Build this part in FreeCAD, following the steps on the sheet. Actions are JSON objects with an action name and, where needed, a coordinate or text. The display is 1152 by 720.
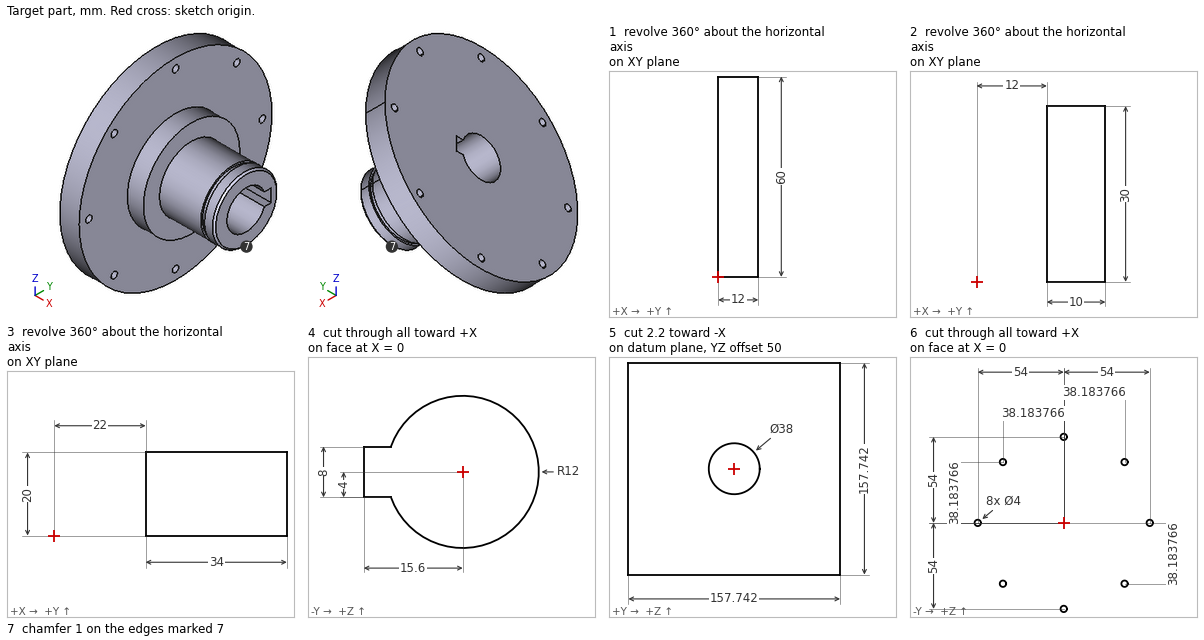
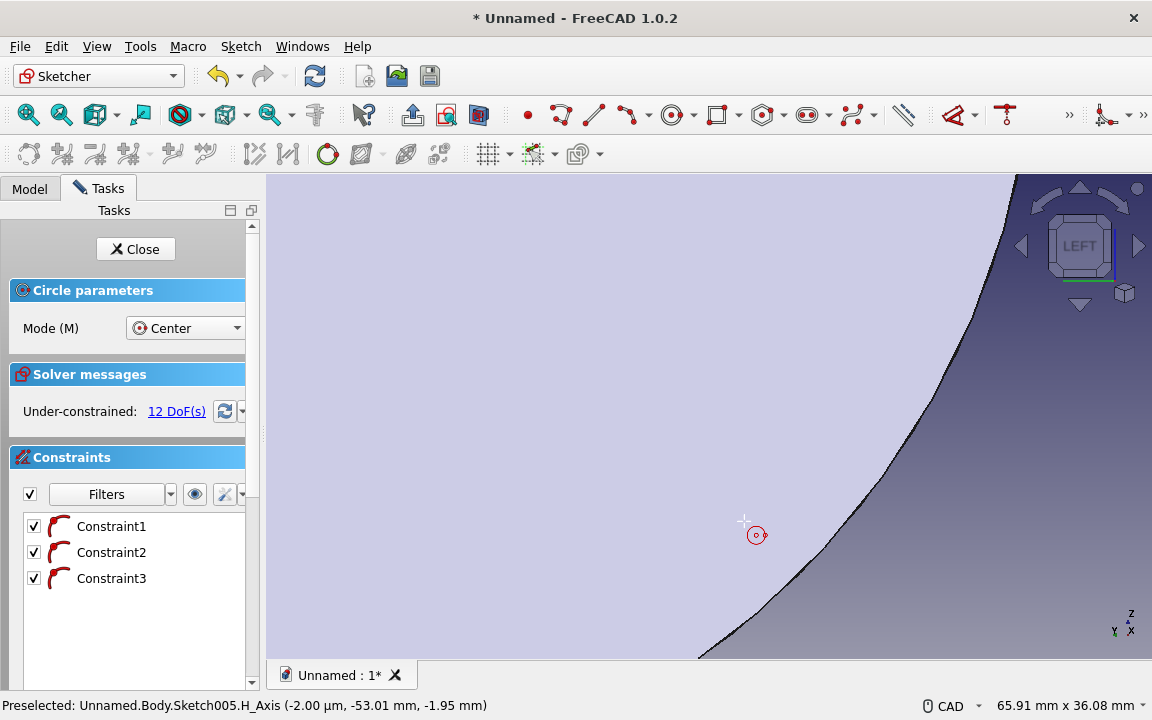
{"action": "scroll", "coordinate": [744, 521], "scroll_direction": "down", "scroll_amount": 8}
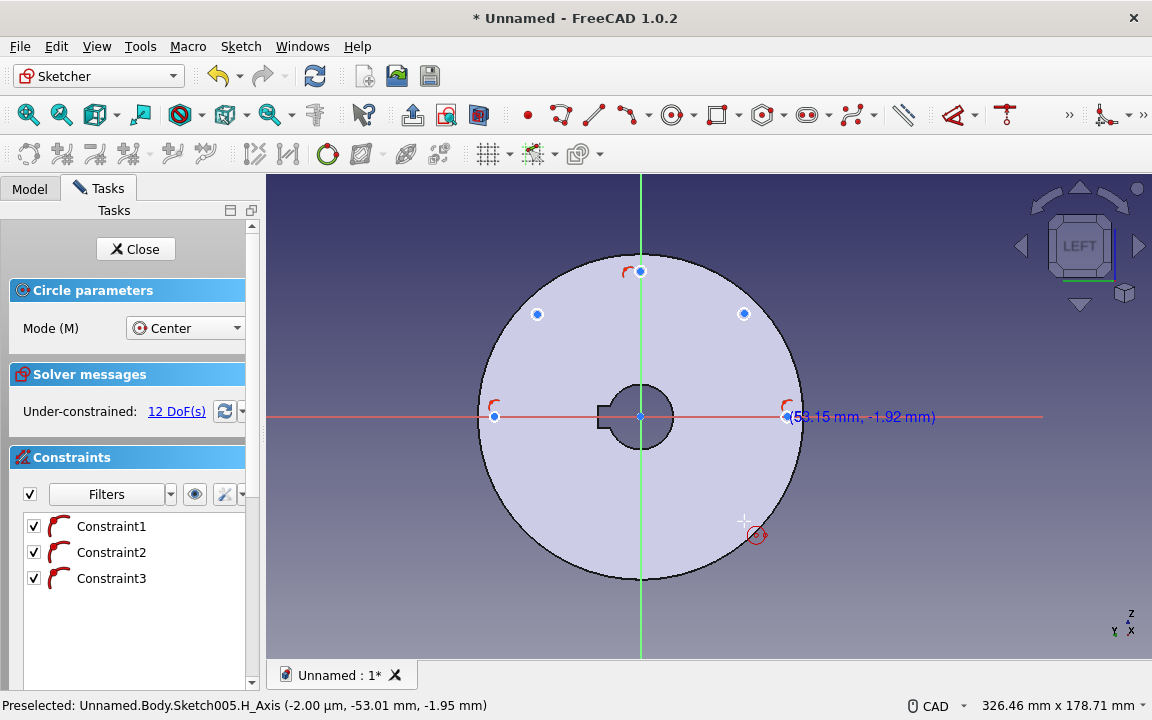
{"action": "left_click", "coordinate": [744, 521]}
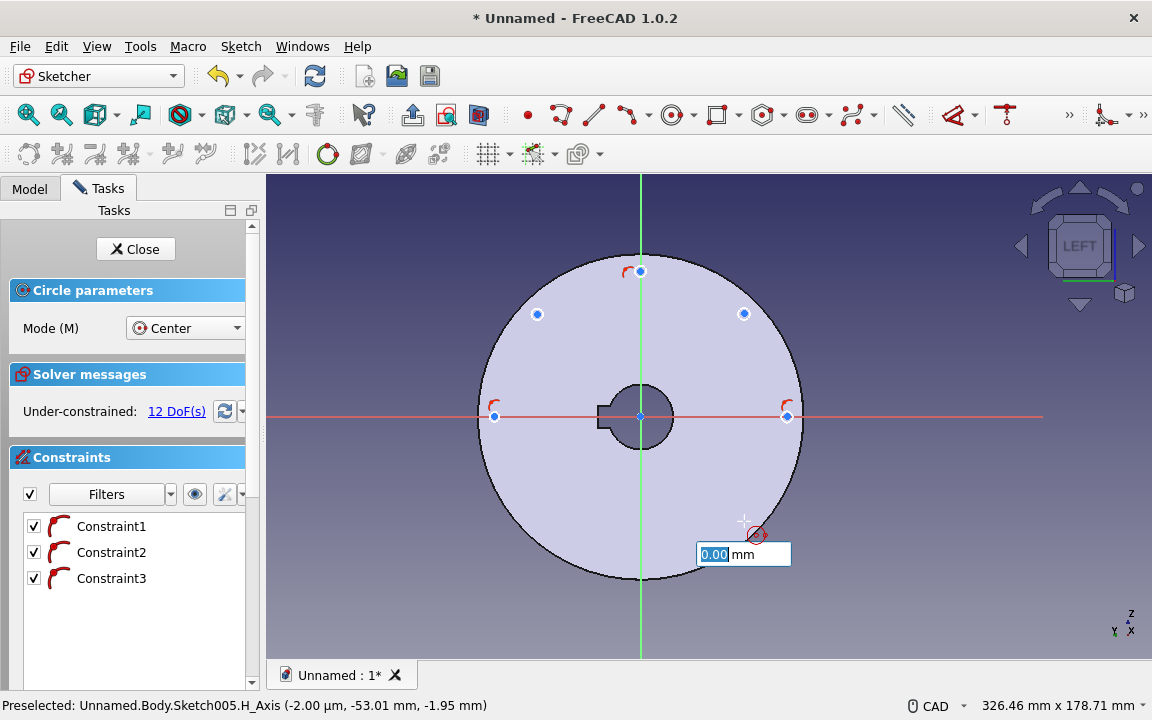
{"action": "scroll", "coordinate": [748, 517], "scroll_direction": "up", "scroll_amount": 6}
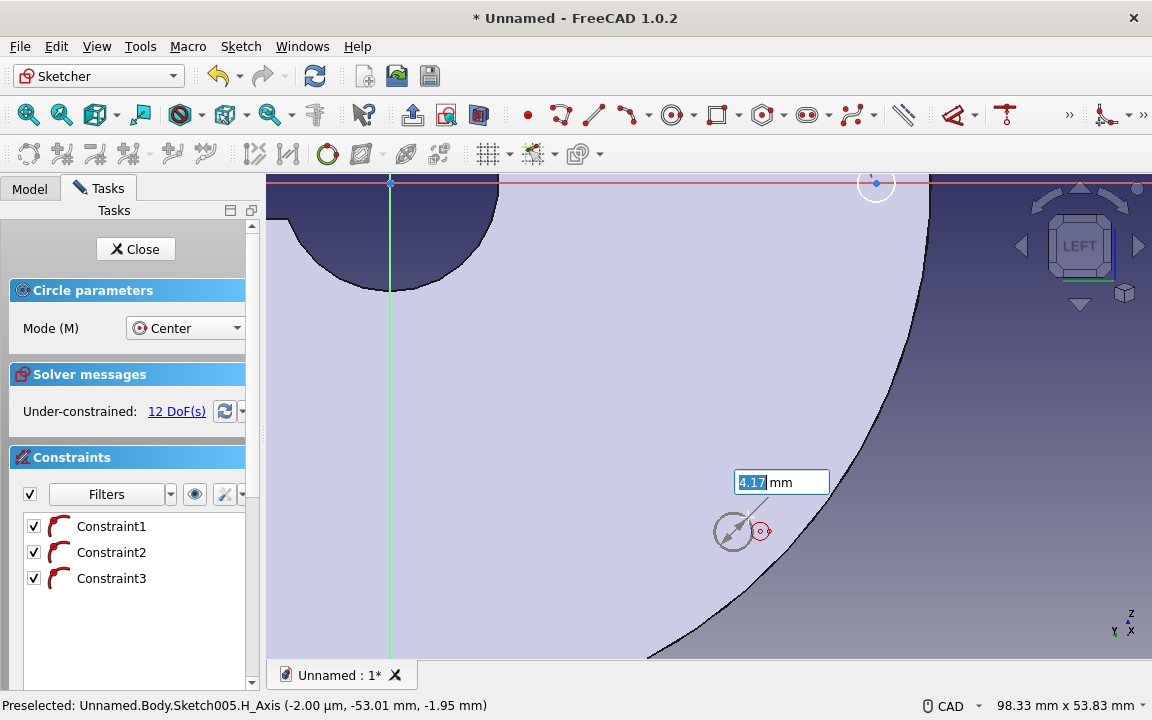
{"action": "left_click", "coordinate": [747, 515]}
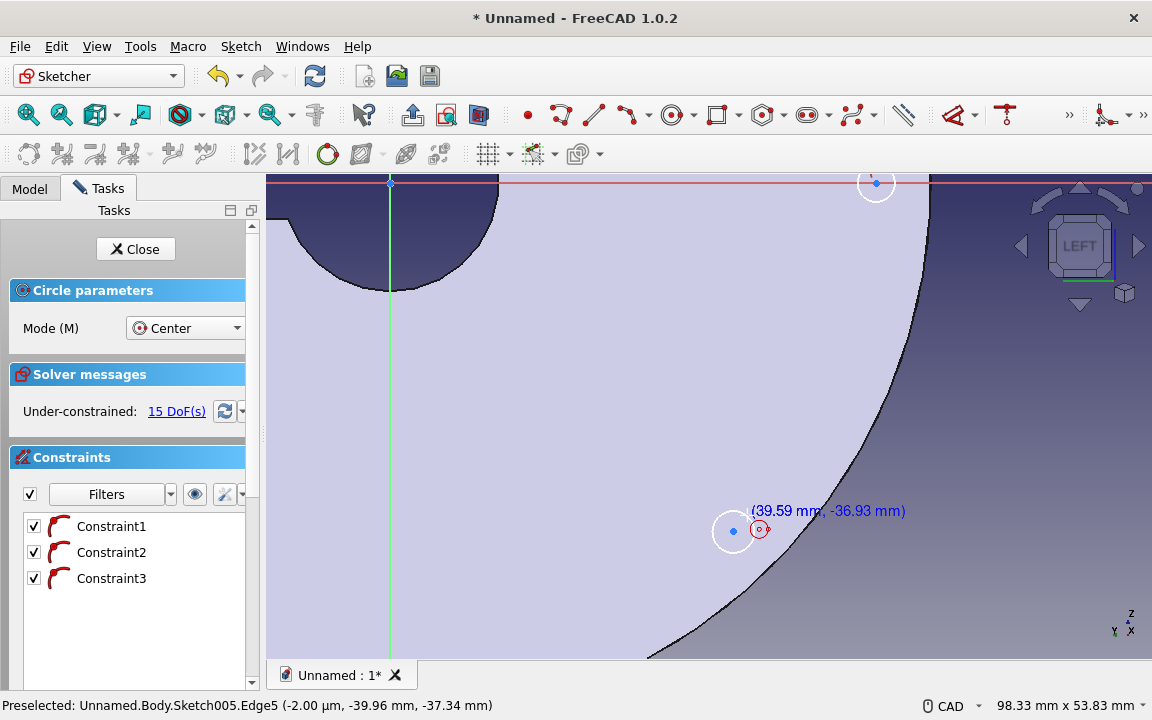
{"action": "scroll", "coordinate": [748, 517], "scroll_direction": "down", "scroll_amount": 6}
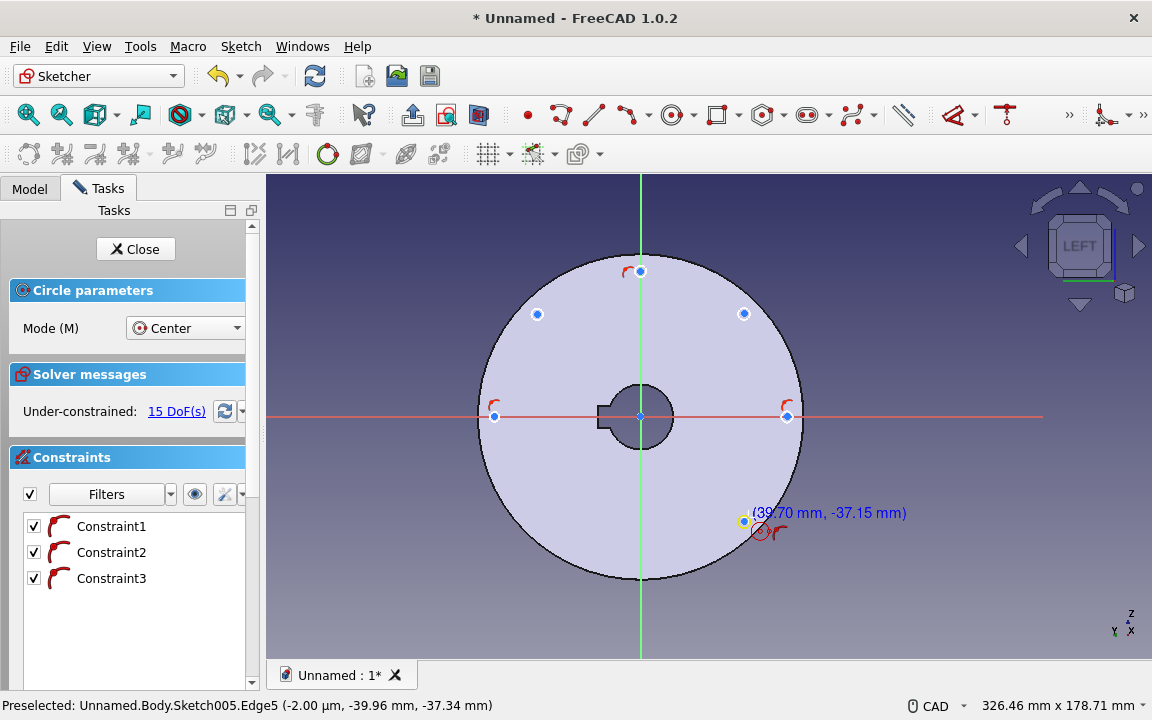
{"action": "scroll", "coordinate": [641, 564], "scroll_direction": "up", "scroll_amount": 8}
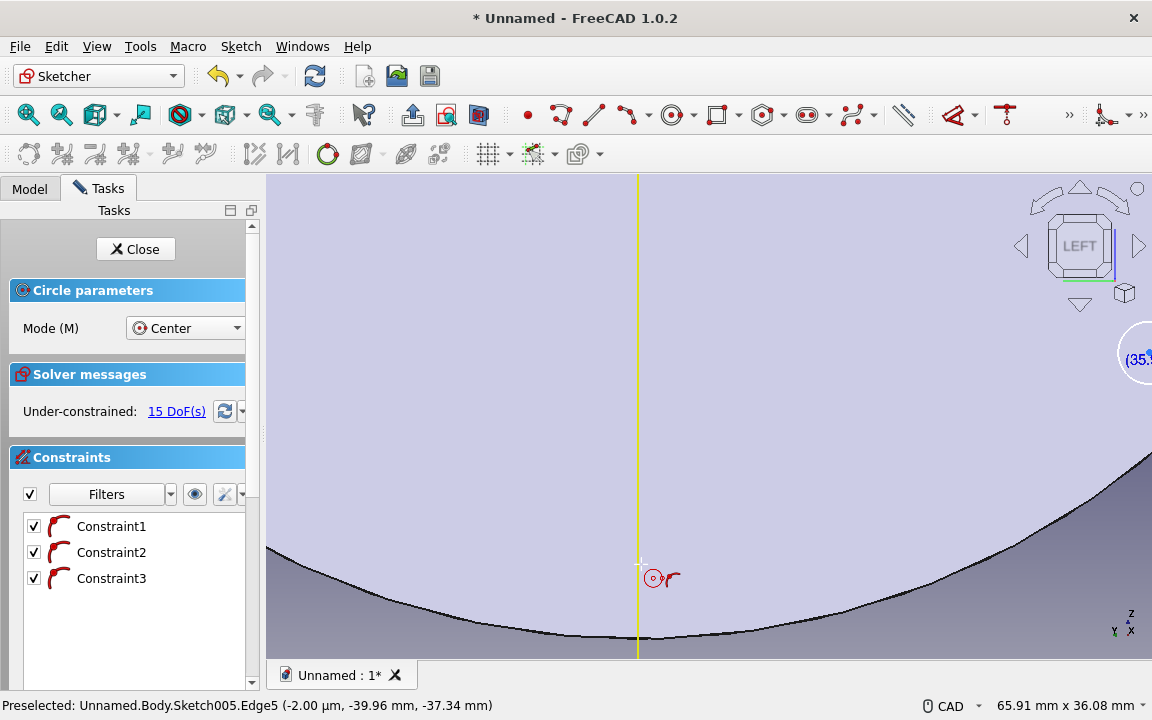
{"action": "scroll", "coordinate": [641, 564], "scroll_direction": "down", "scroll_amount": 8}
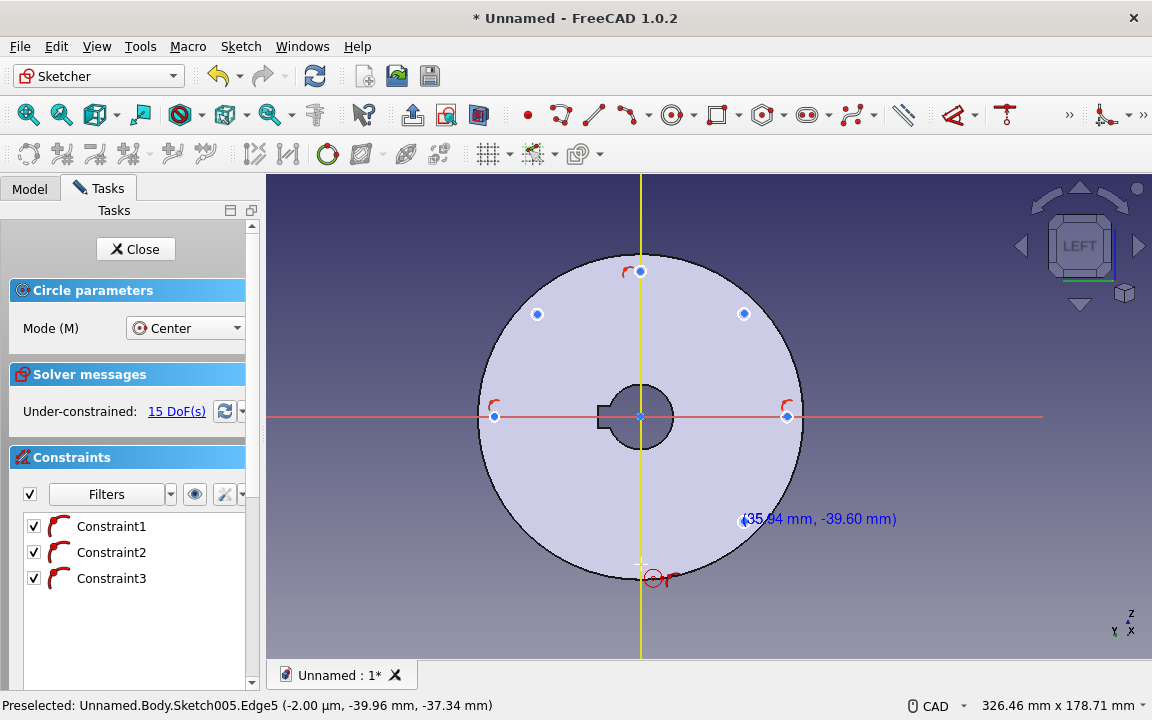
{"action": "left_click", "coordinate": [641, 564]}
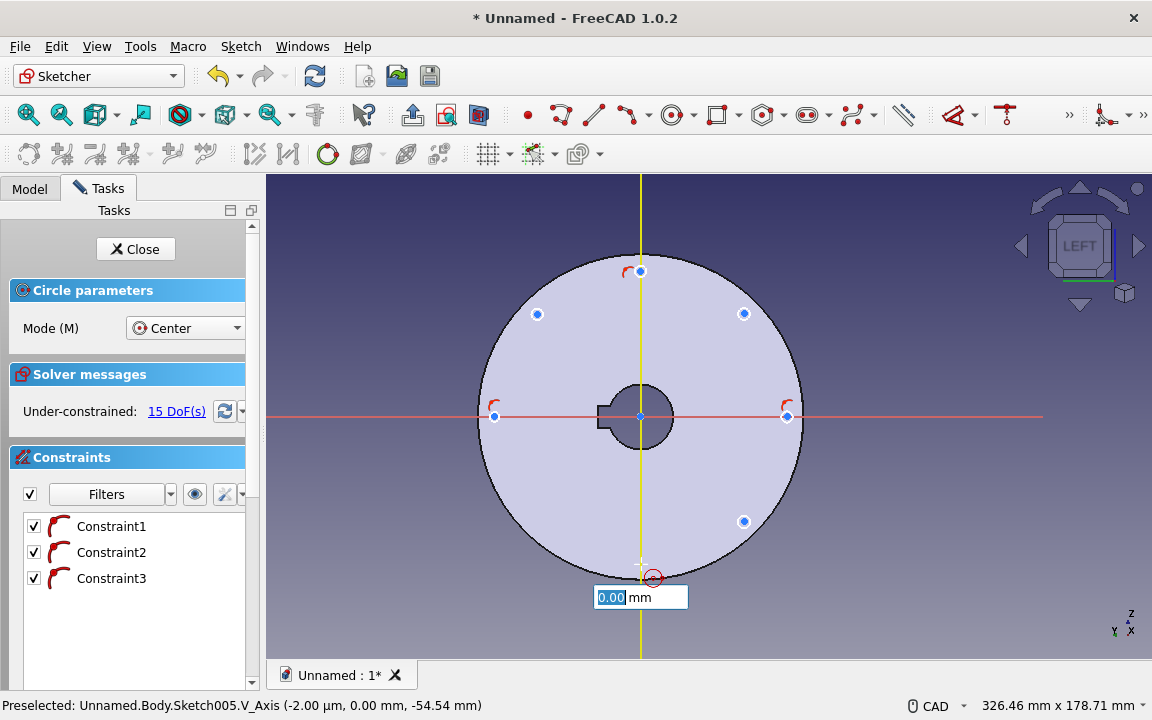
{"action": "scroll", "coordinate": [646, 562], "scroll_direction": "up", "scroll_amount": 6}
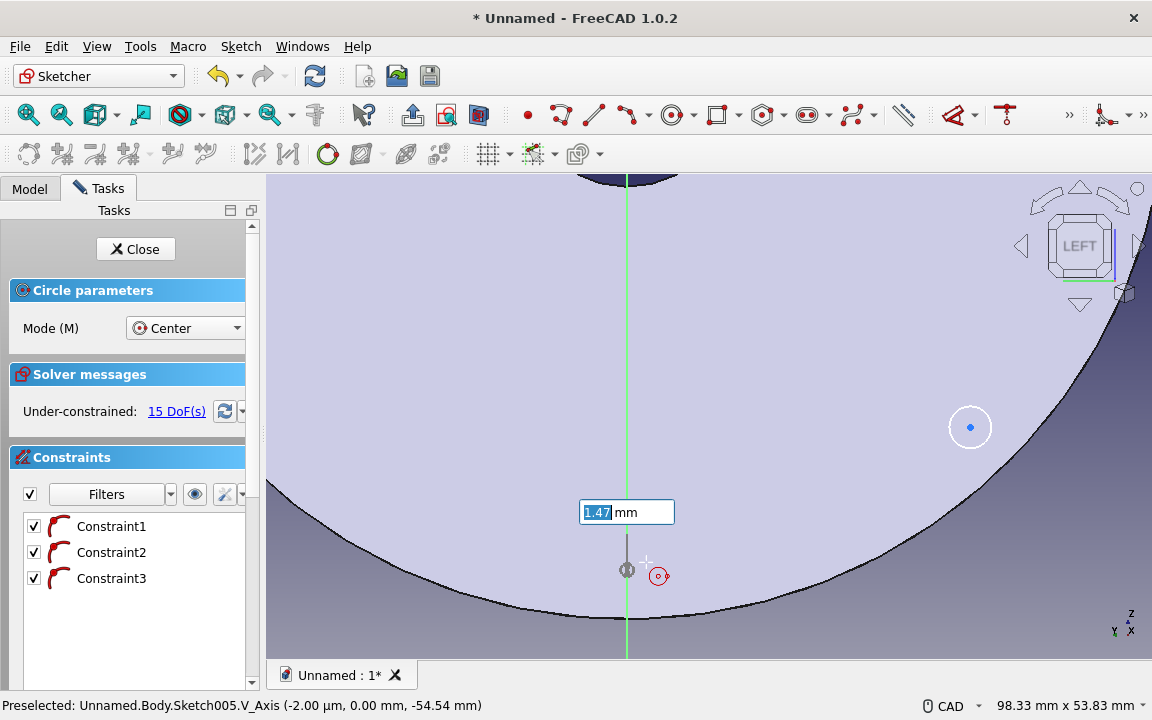
{"action": "left_click", "coordinate": [644, 559]}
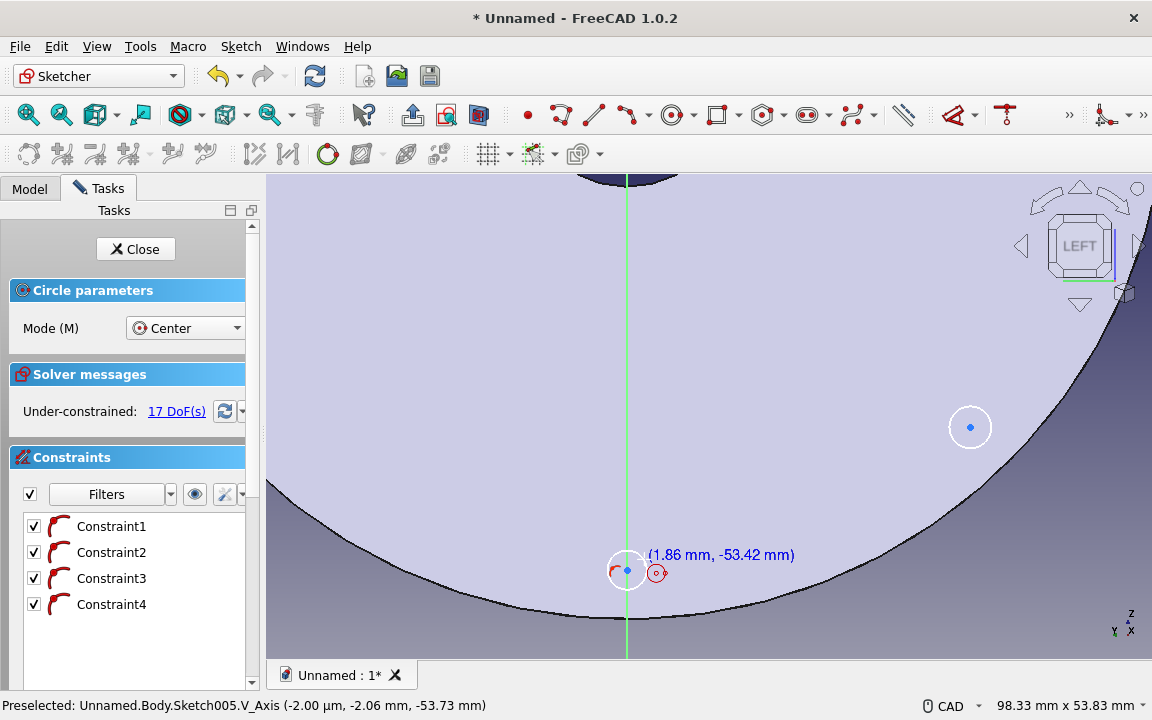
{"action": "scroll", "coordinate": [646, 562], "scroll_direction": "down", "scroll_amount": 6}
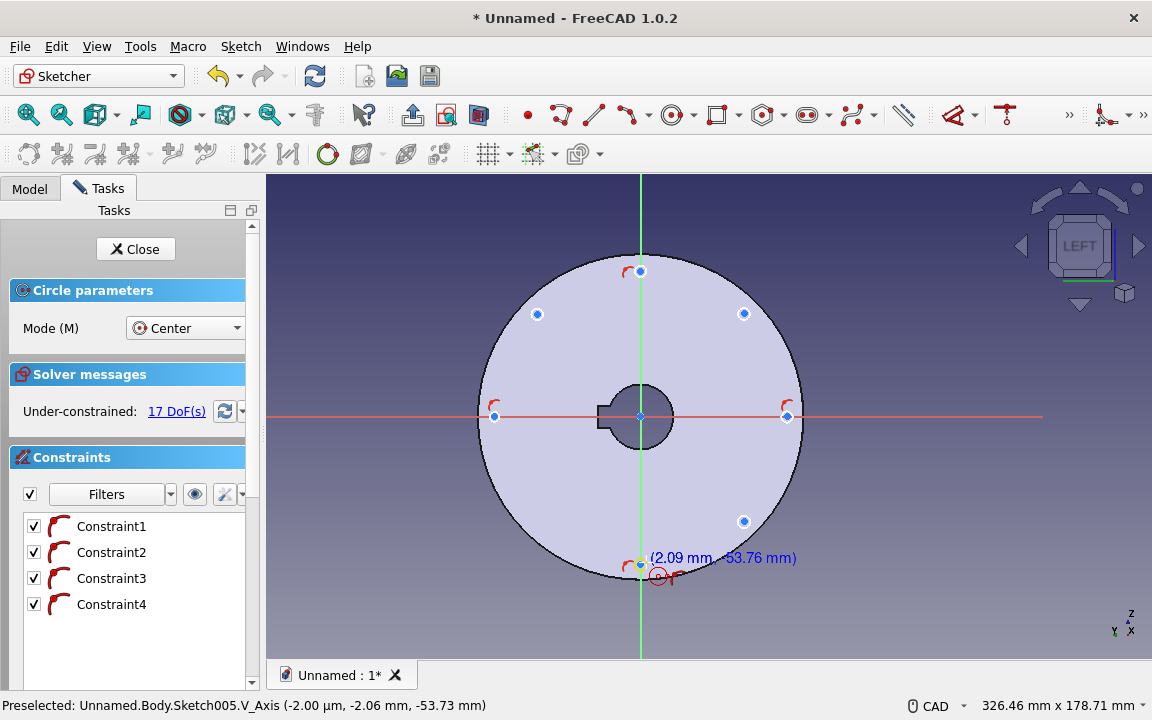
{"action": "scroll", "coordinate": [537, 521], "scroll_direction": "up", "scroll_amount": 8}